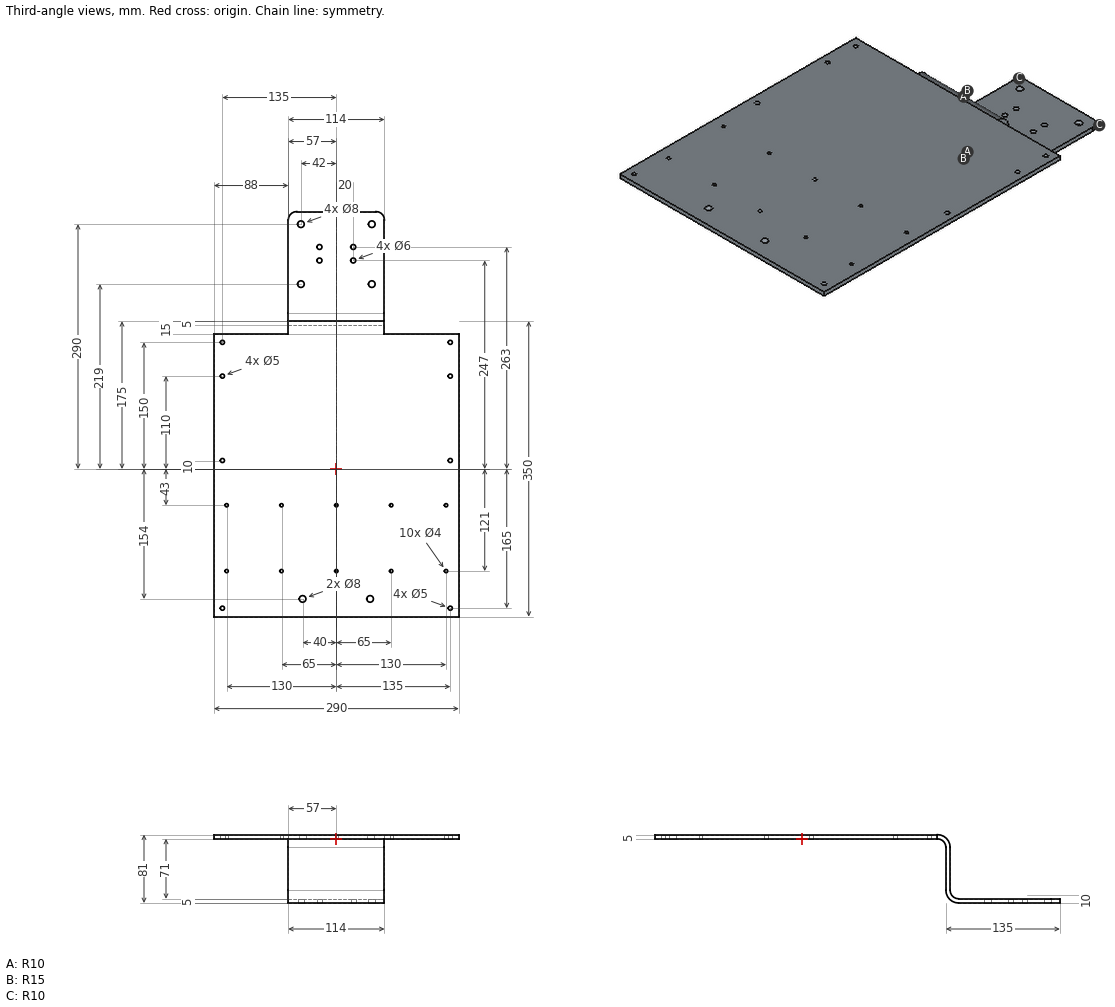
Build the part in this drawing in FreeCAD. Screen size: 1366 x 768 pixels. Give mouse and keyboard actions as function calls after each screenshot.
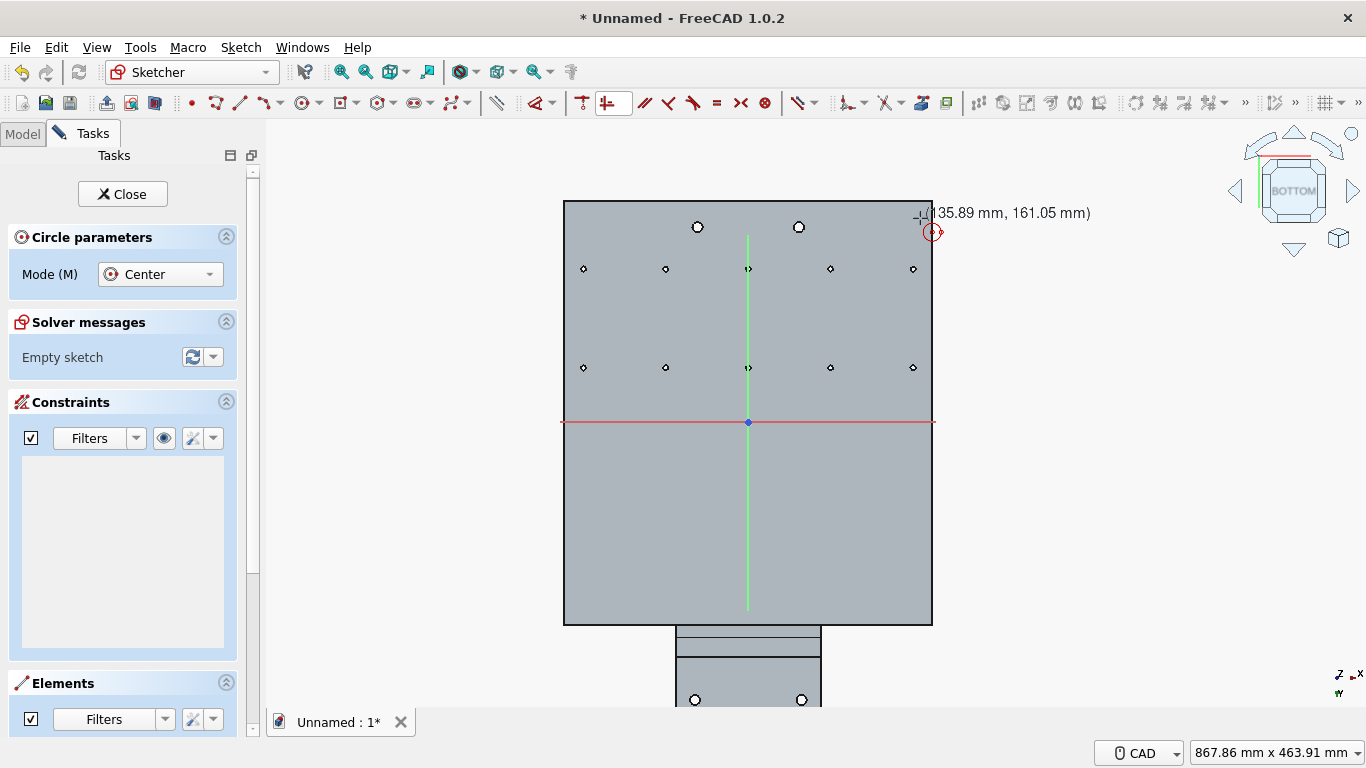
click(919, 213)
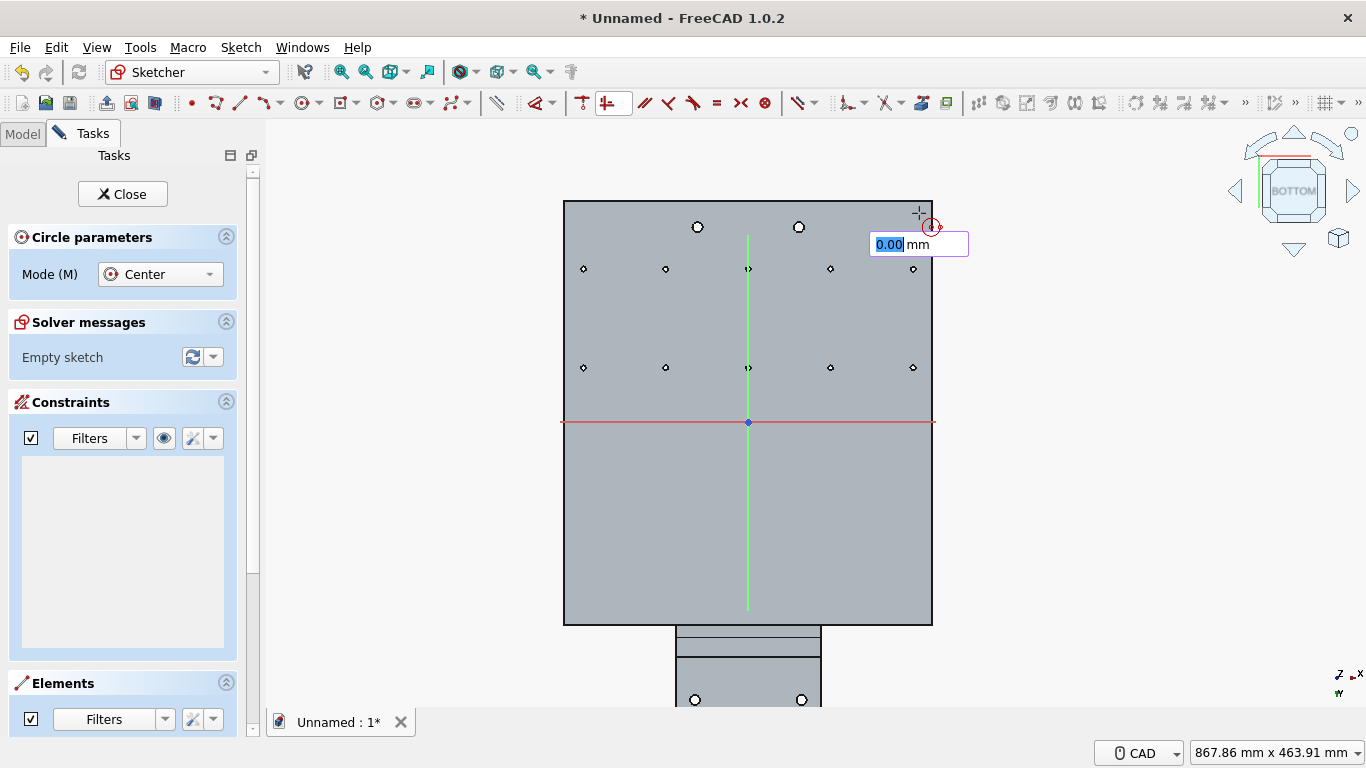
scroll(922, 211, up, 9)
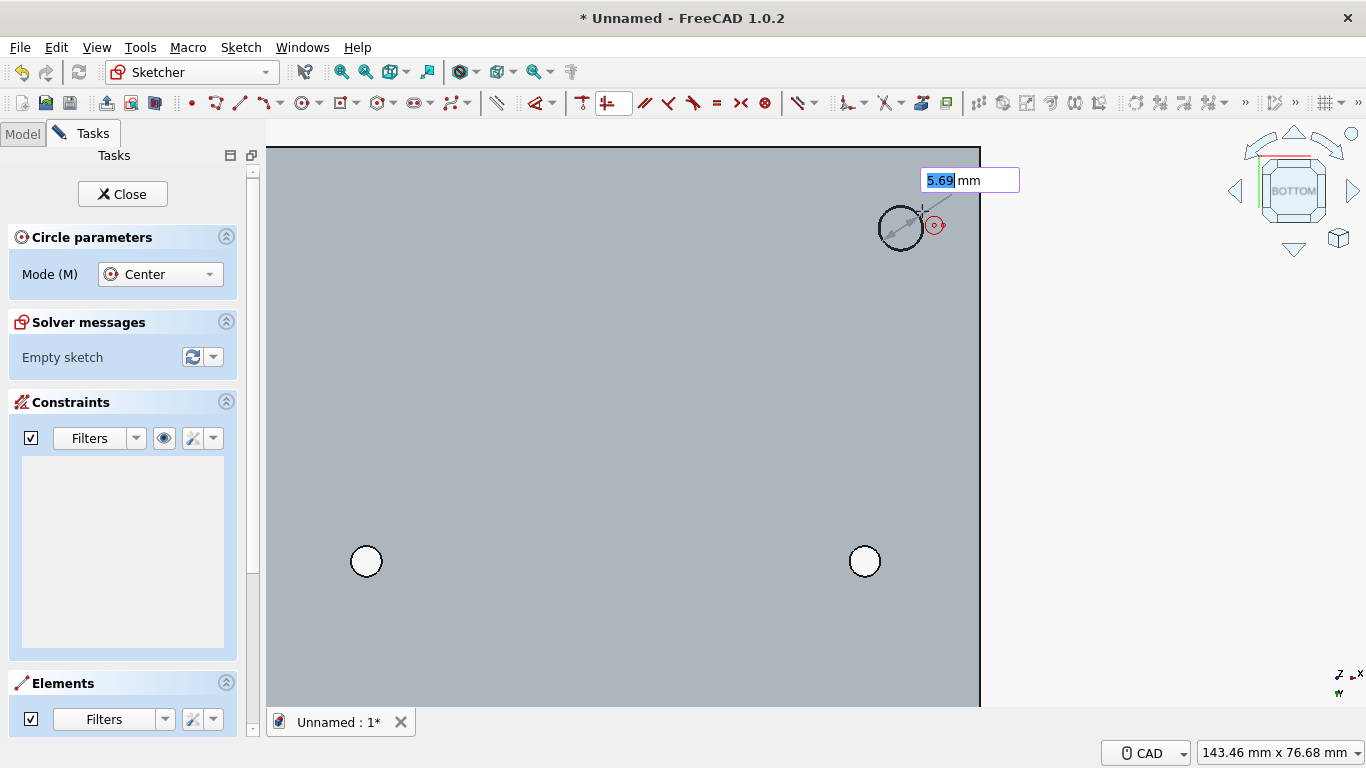
click(917, 210)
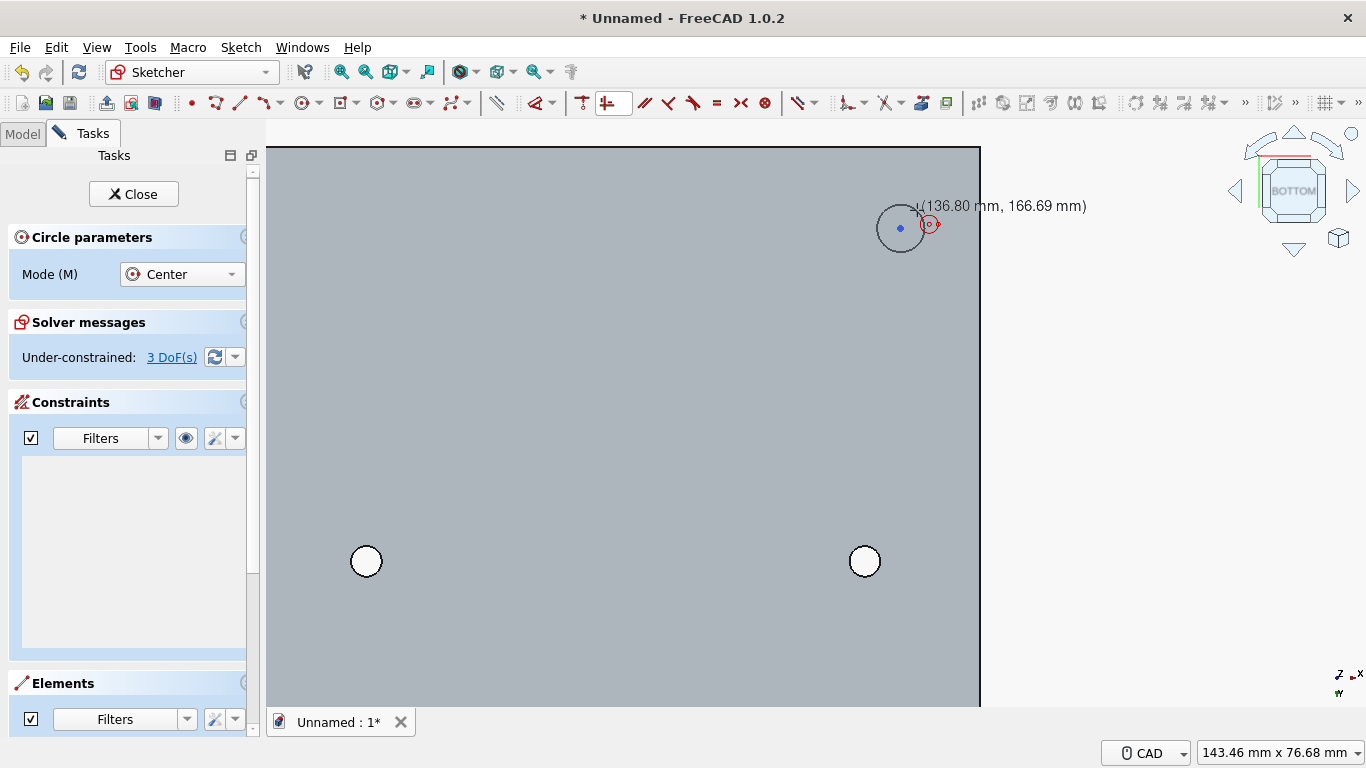
scroll(922, 211, down, 9)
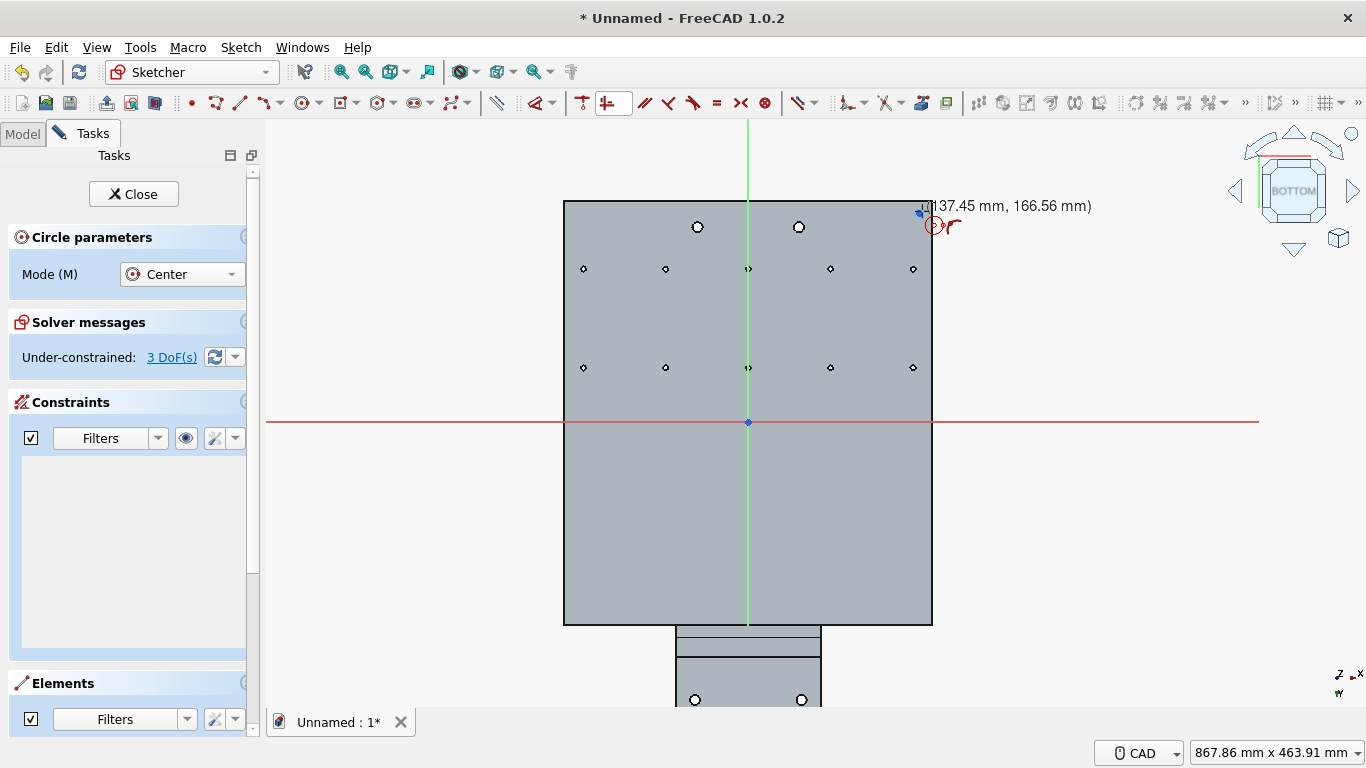
scroll(577, 213, up, 10)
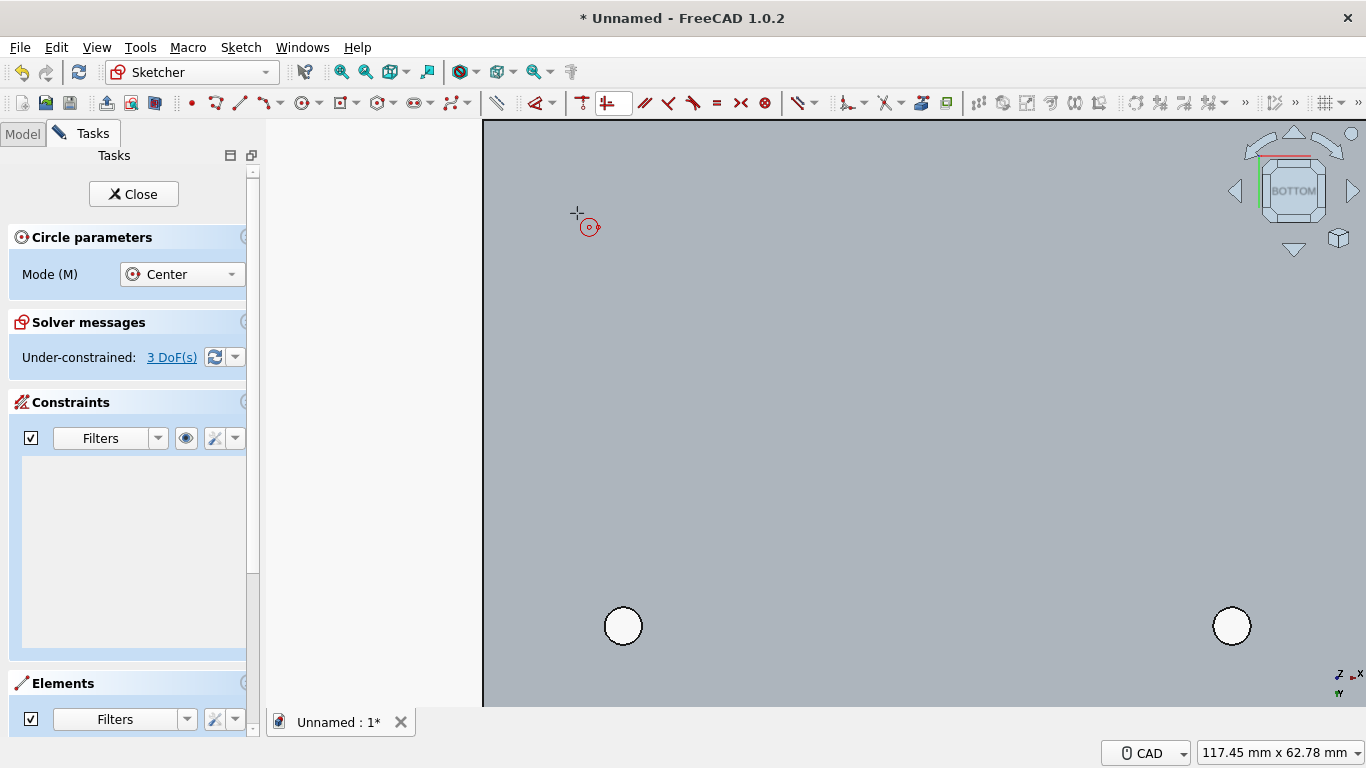
scroll(576, 213, down, 10)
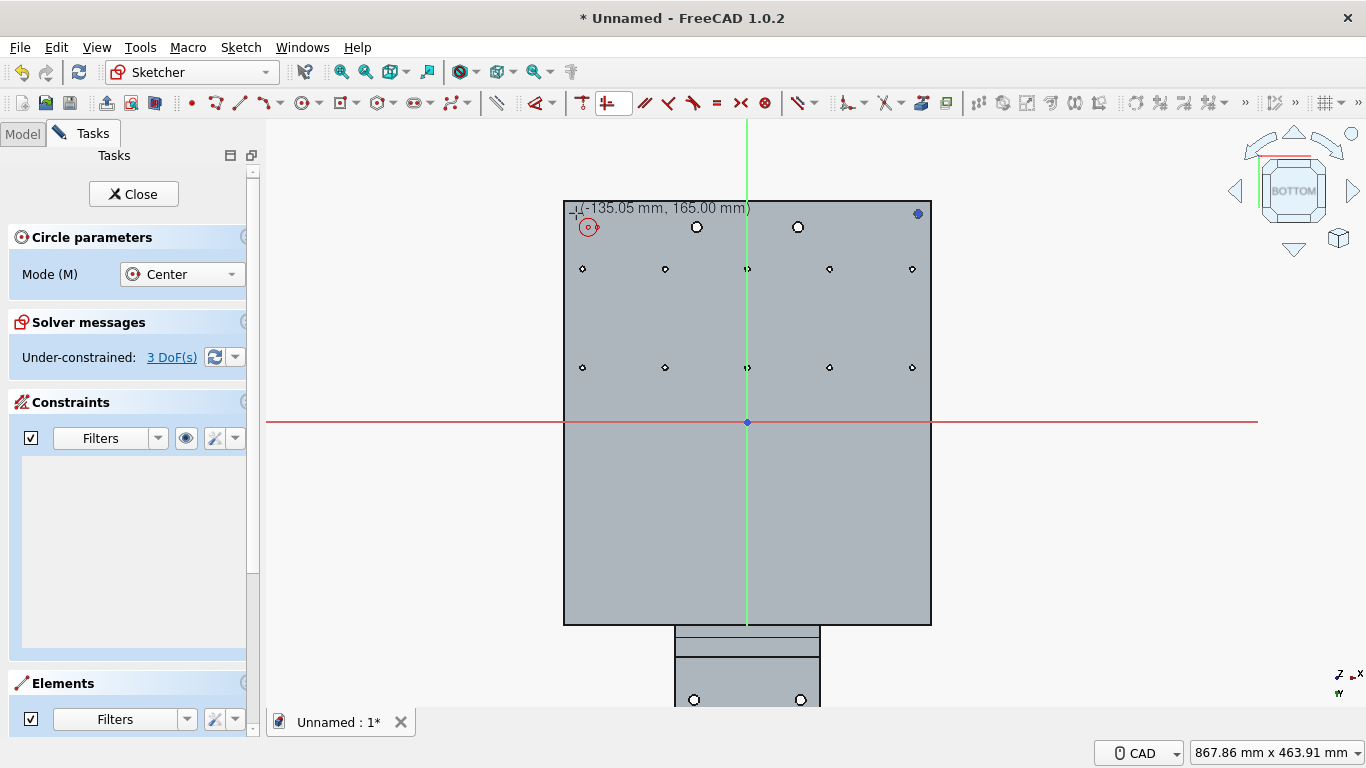
click(576, 213)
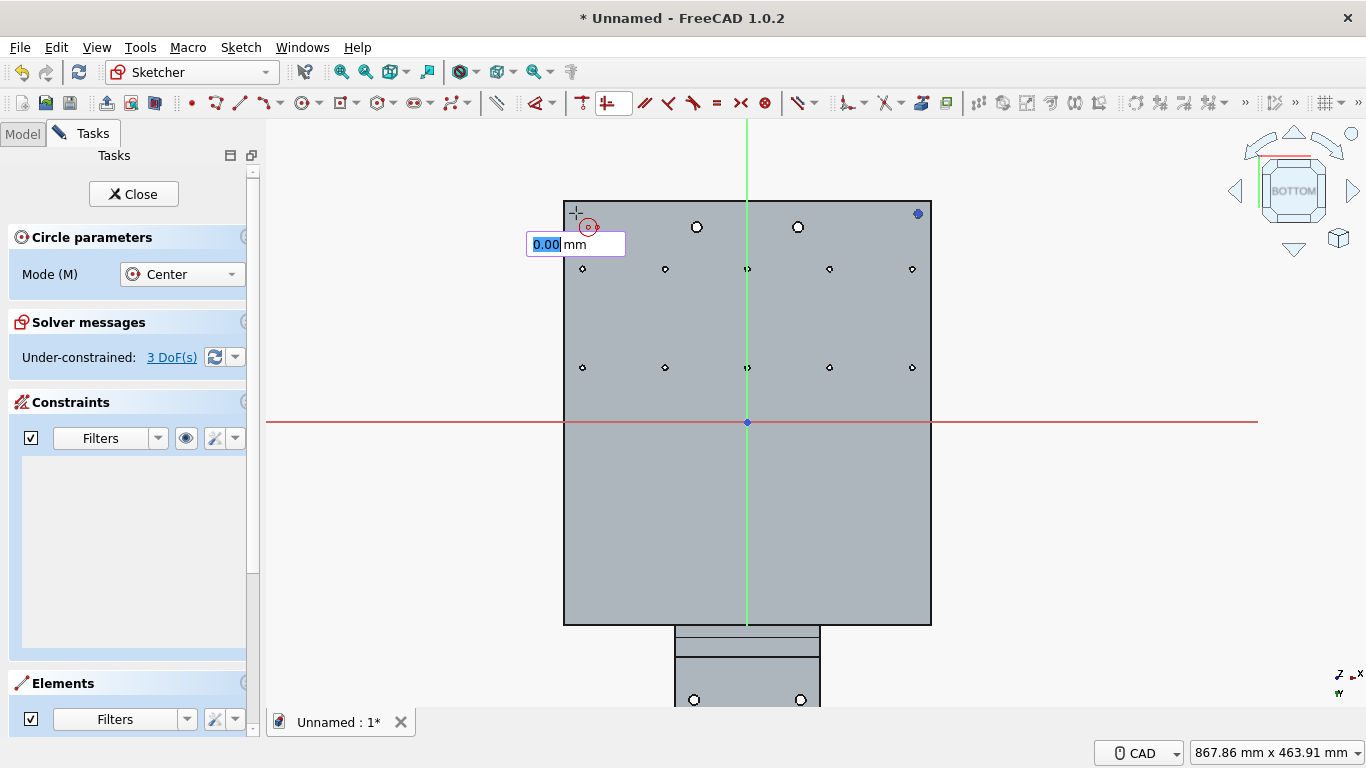
scroll(579, 211, up, 9)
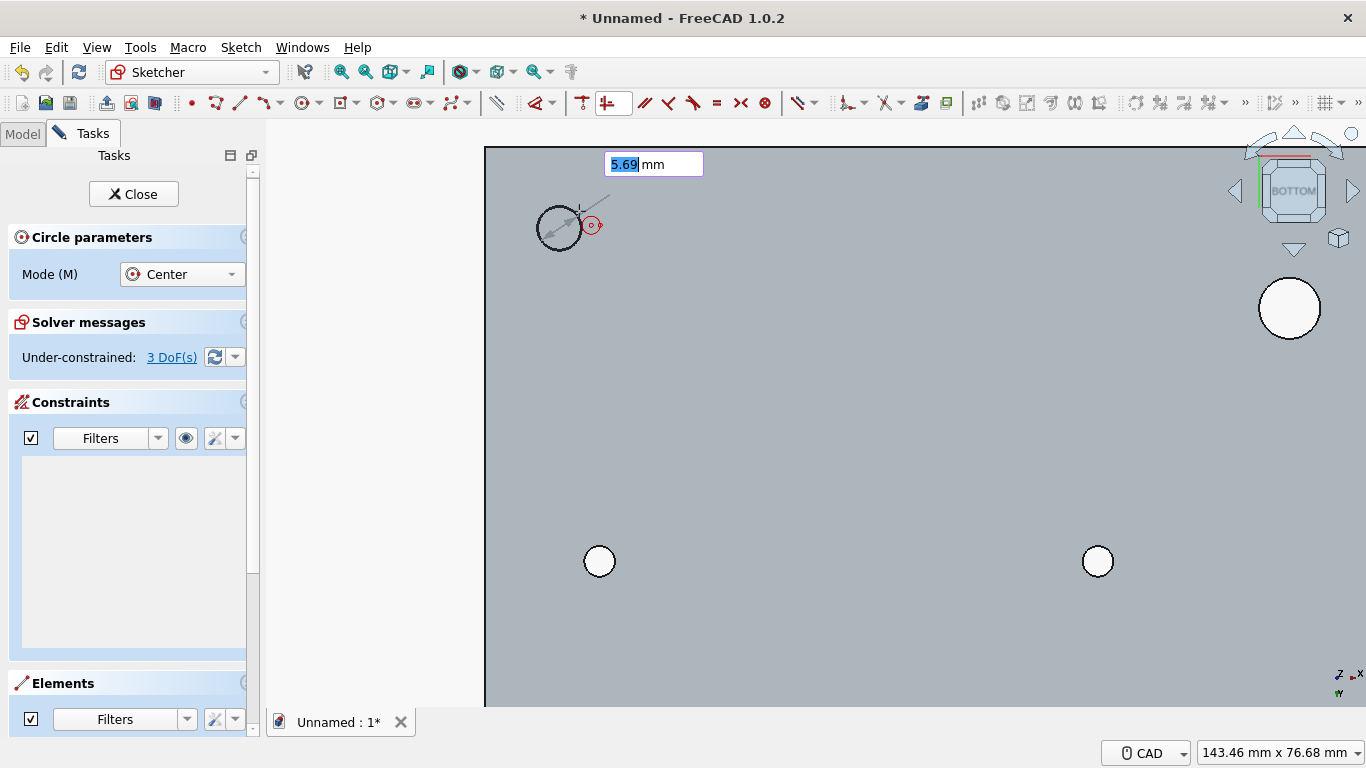
click(575, 210)